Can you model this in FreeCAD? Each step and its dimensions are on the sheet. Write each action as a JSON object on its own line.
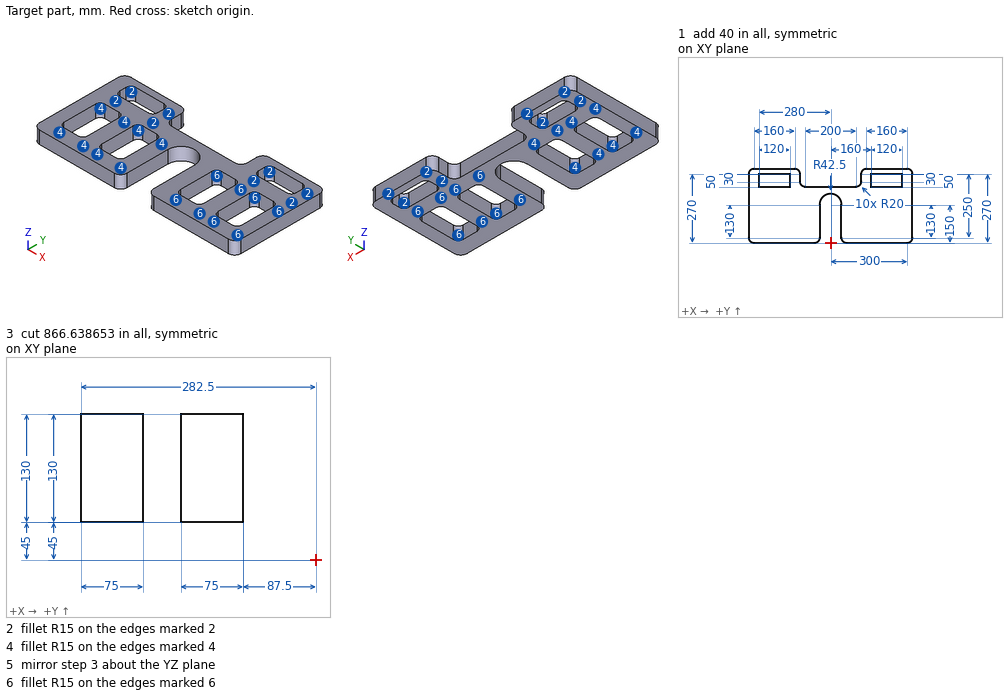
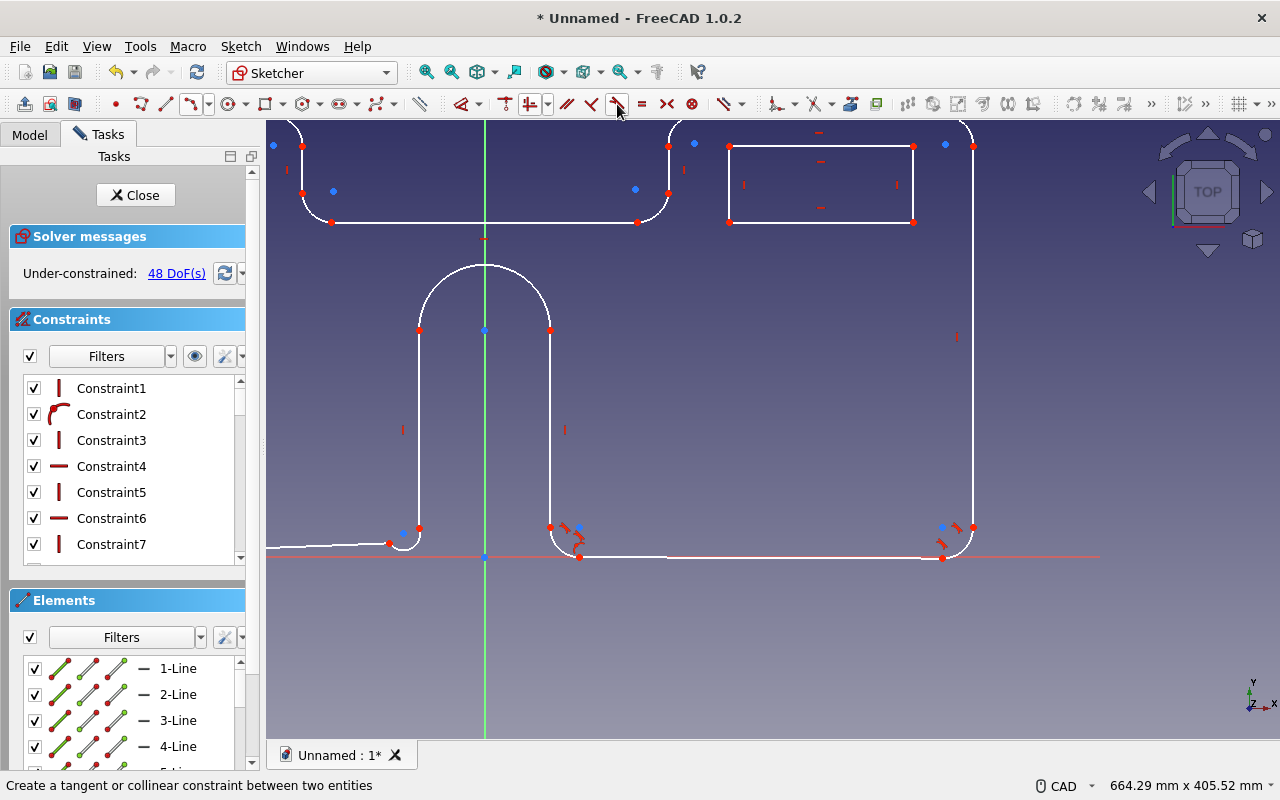
{"action": "left_click", "coordinate": [973, 413]}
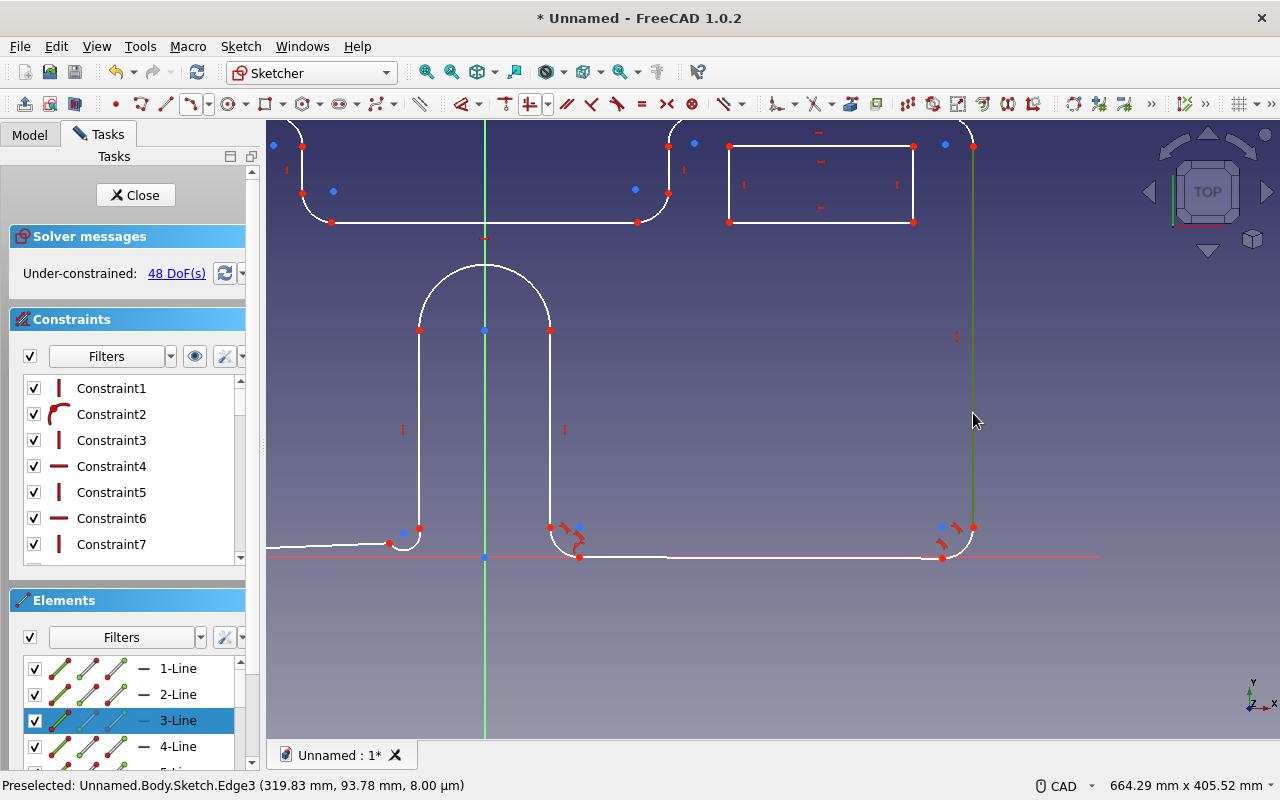
{"action": "scroll", "coordinate": [972, 543], "scroll_direction": "down", "scroll_amount": 3}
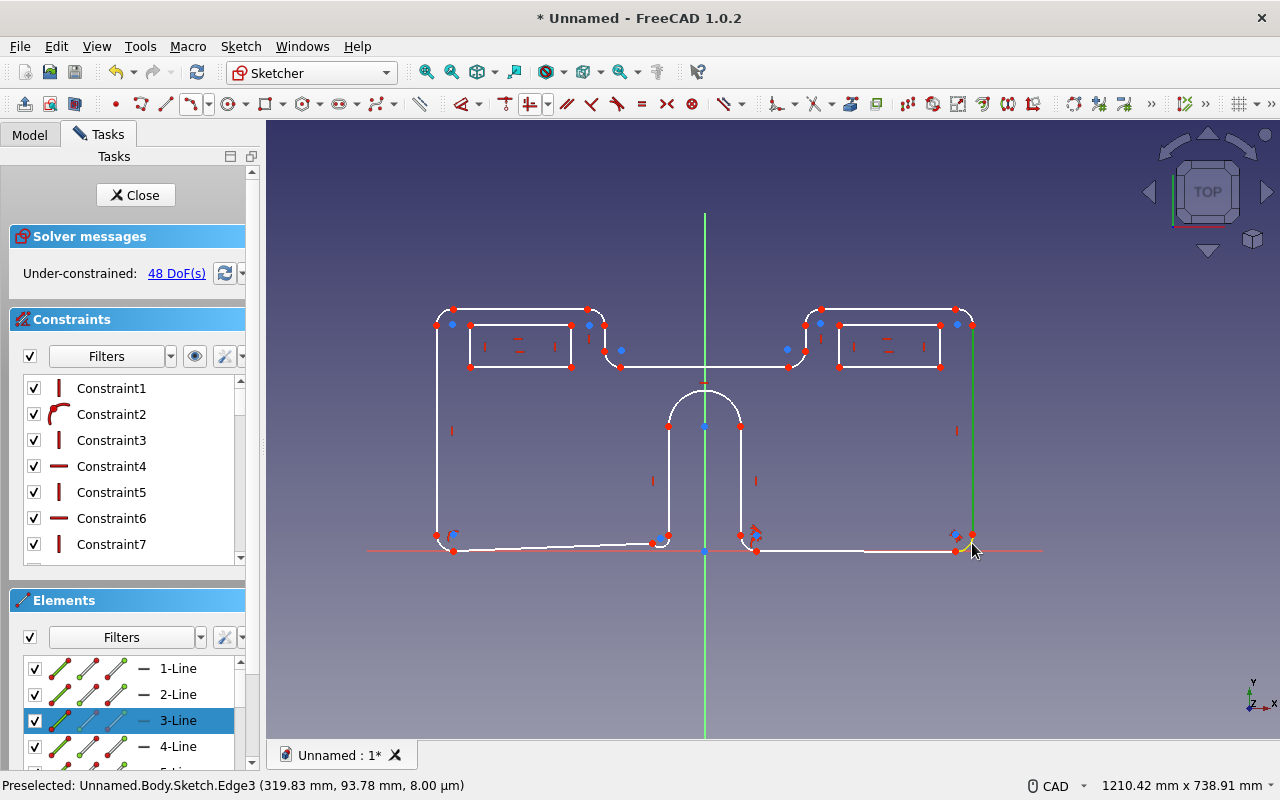
{"action": "scroll", "coordinate": [971, 318], "scroll_direction": "up", "scroll_amount": 3}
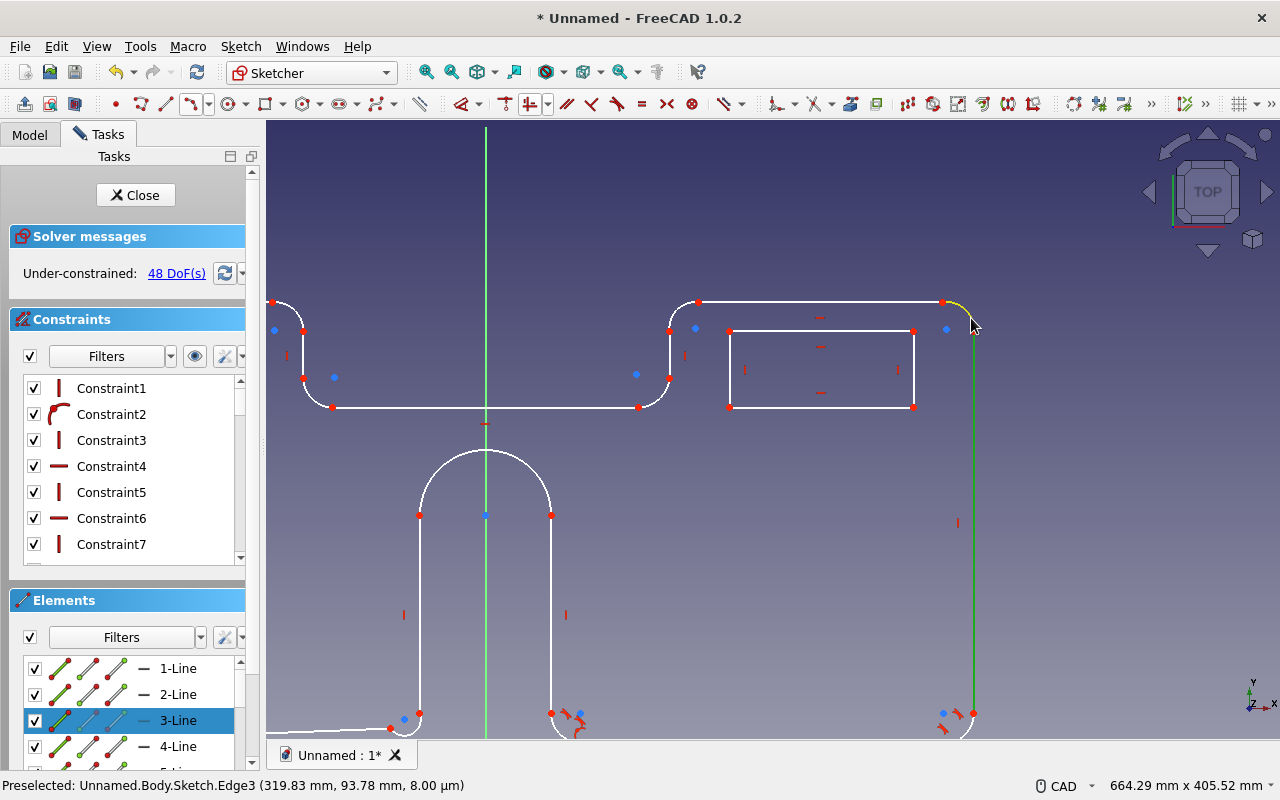
{"action": "left_click", "coordinate": [971, 317]}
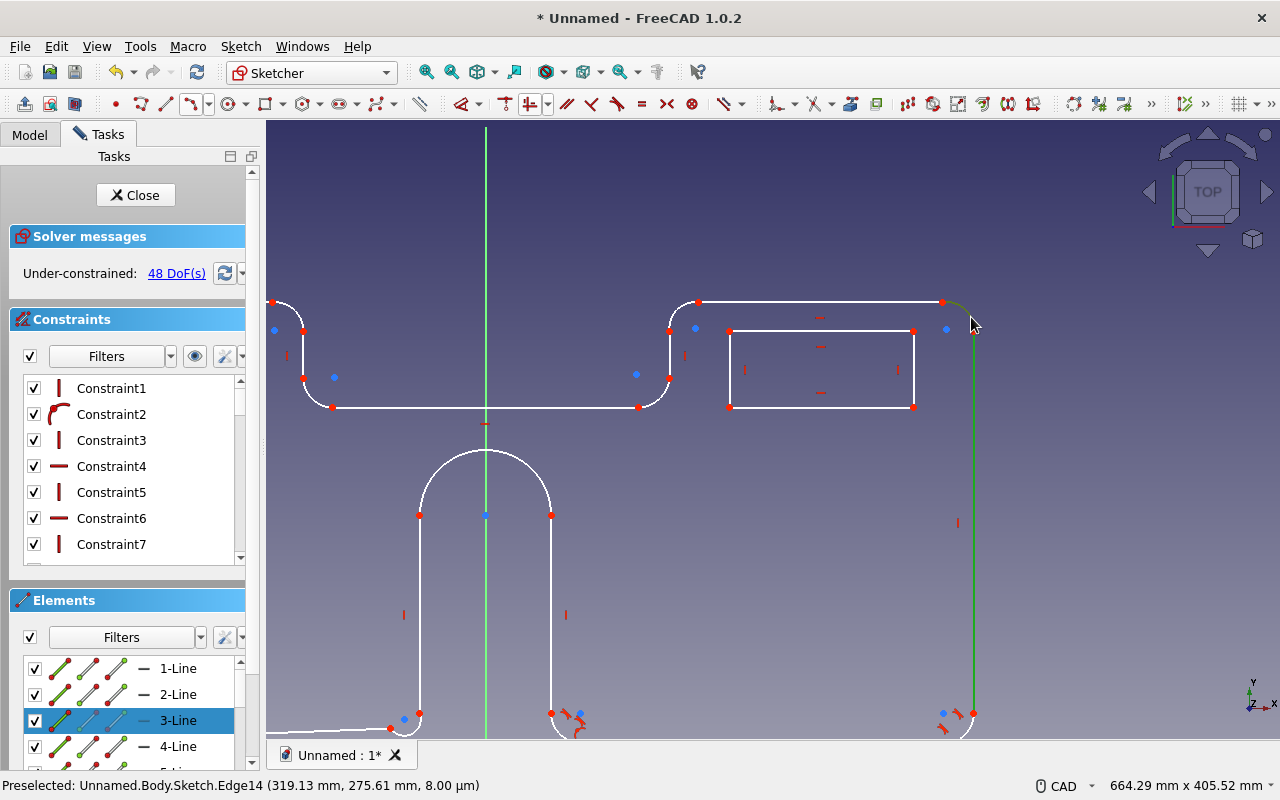
{"action": "left_click", "coordinate": [617, 104]}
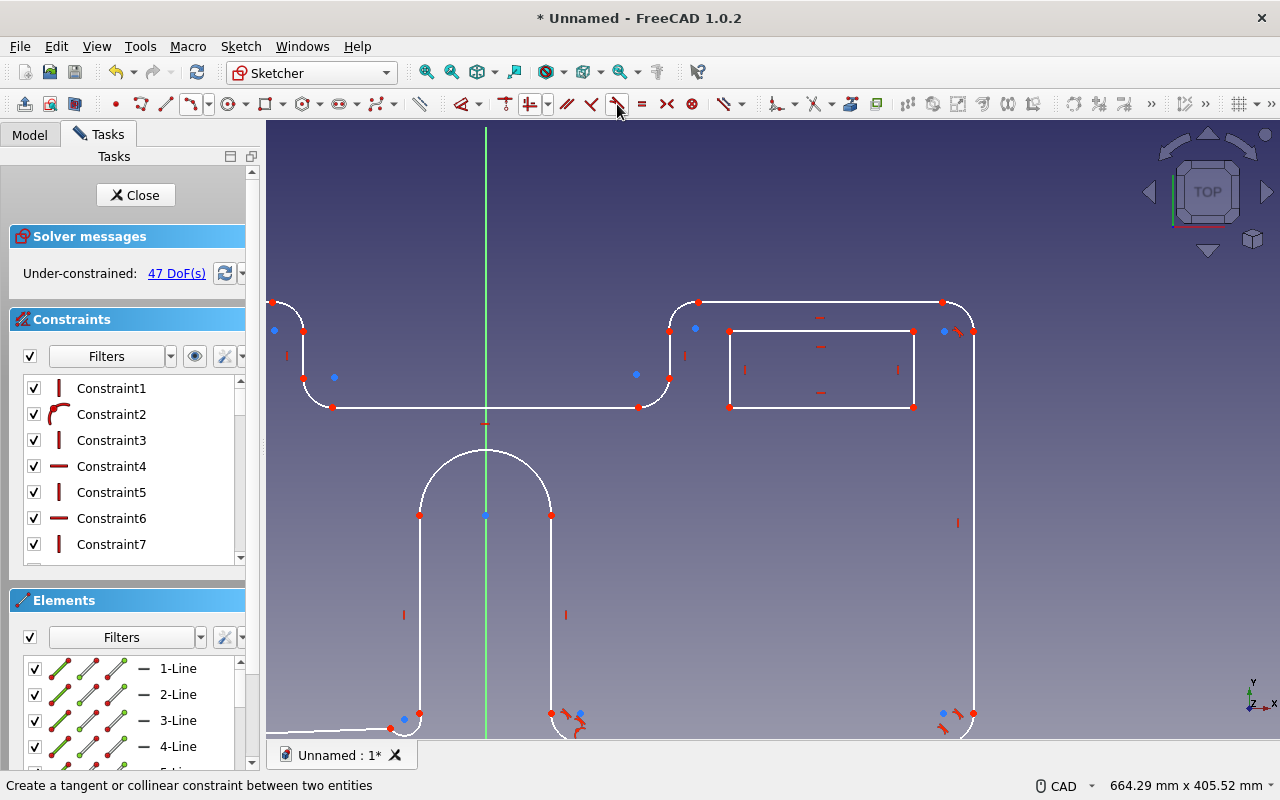
{"action": "left_click", "coordinate": [870, 302]}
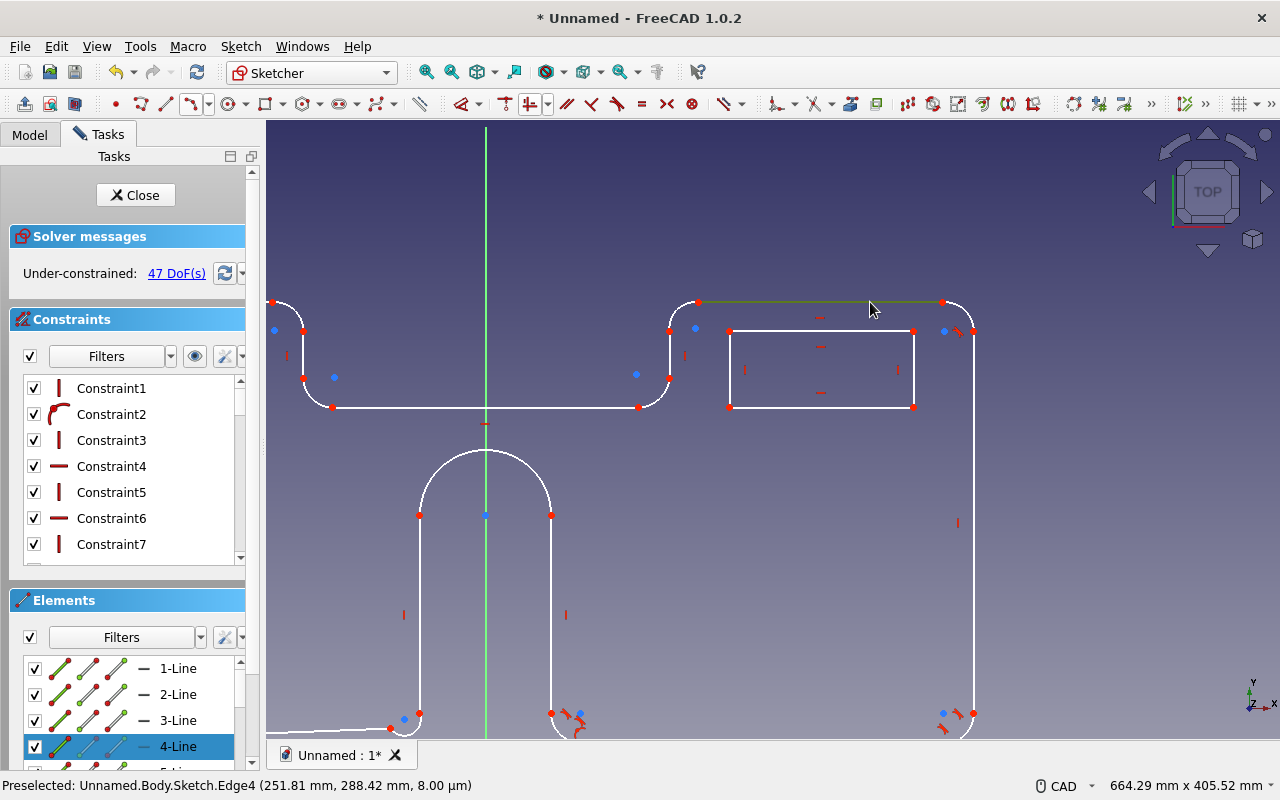
{"action": "left_click", "coordinate": [970, 318]}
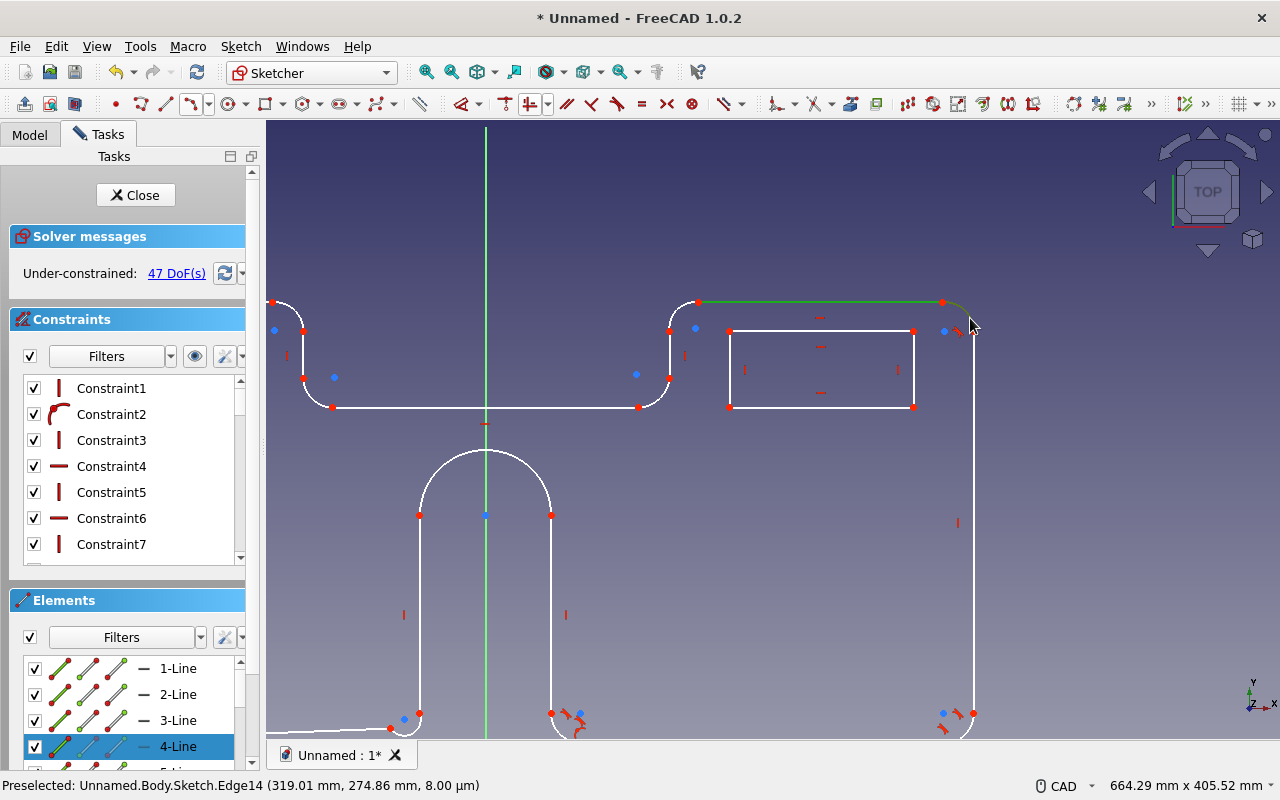
{"action": "key", "text": "t"}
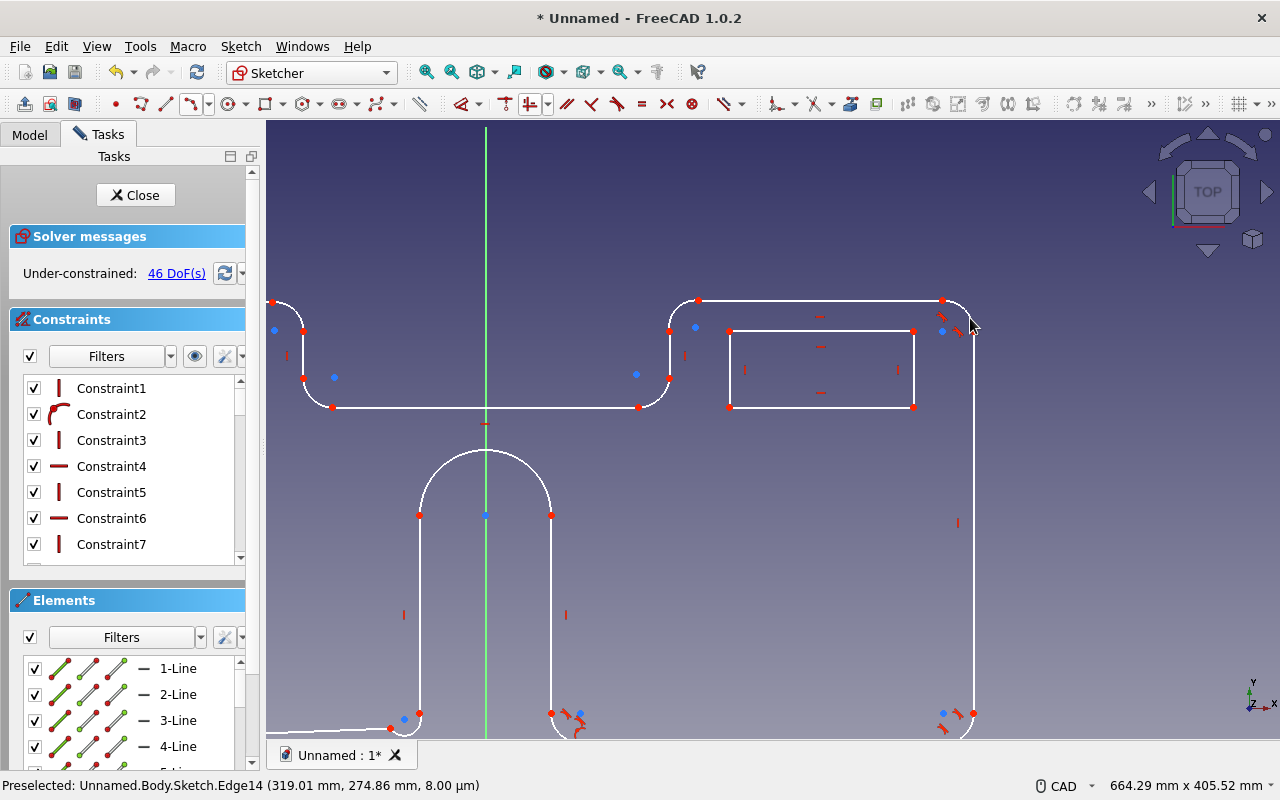
{"action": "left_click", "coordinate": [870, 301]}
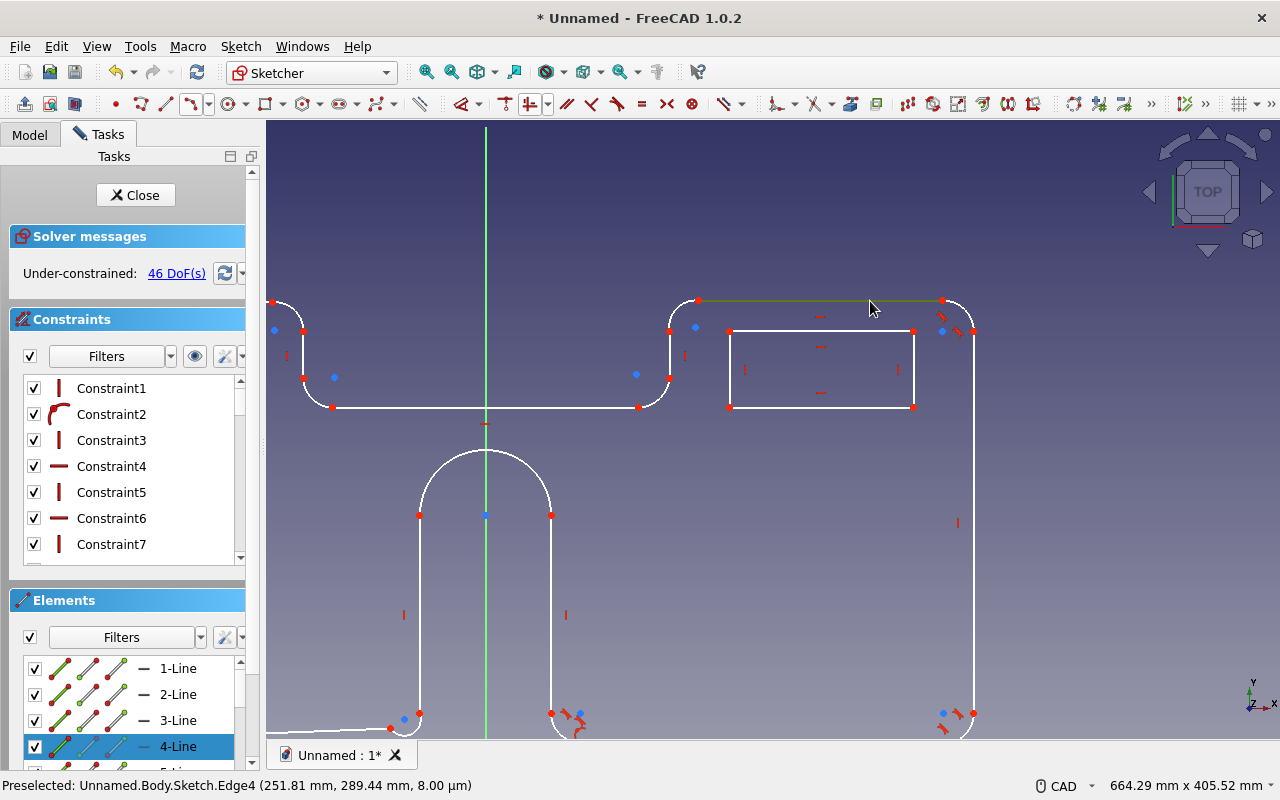
{"action": "left_click", "coordinate": [684, 303]}